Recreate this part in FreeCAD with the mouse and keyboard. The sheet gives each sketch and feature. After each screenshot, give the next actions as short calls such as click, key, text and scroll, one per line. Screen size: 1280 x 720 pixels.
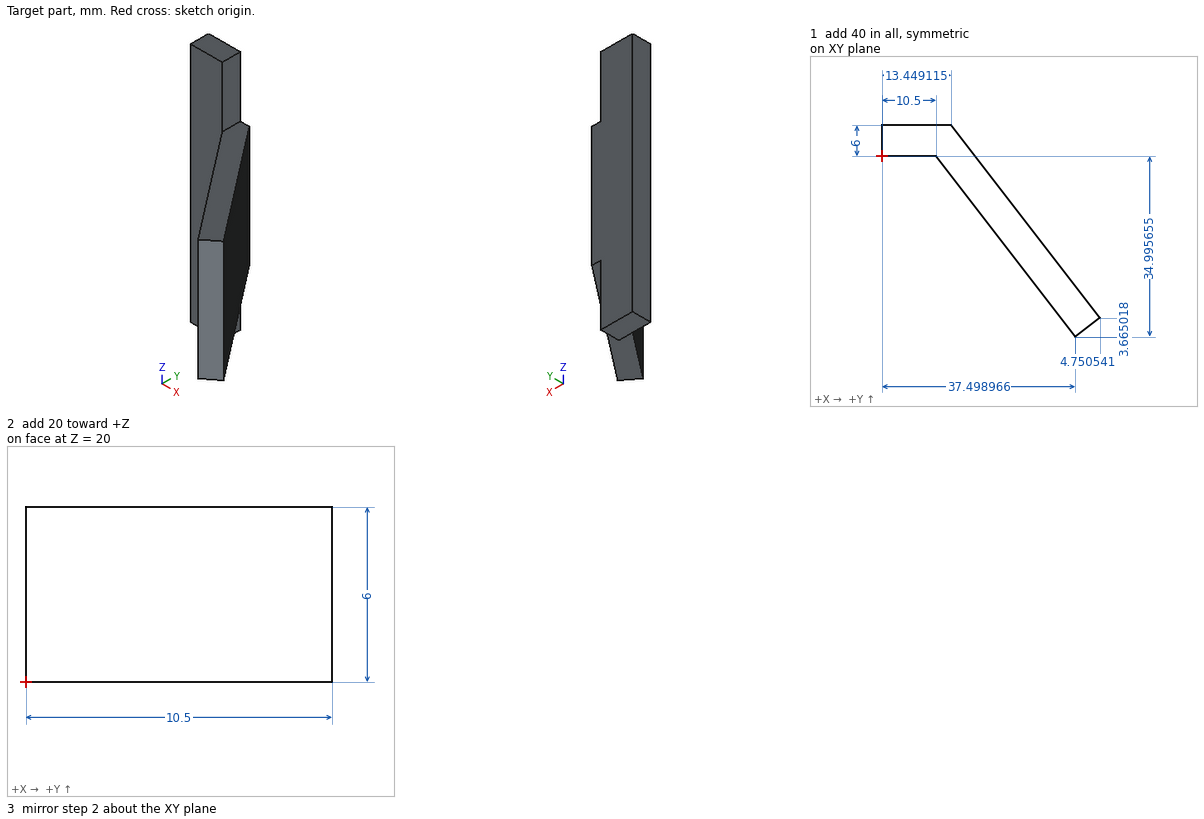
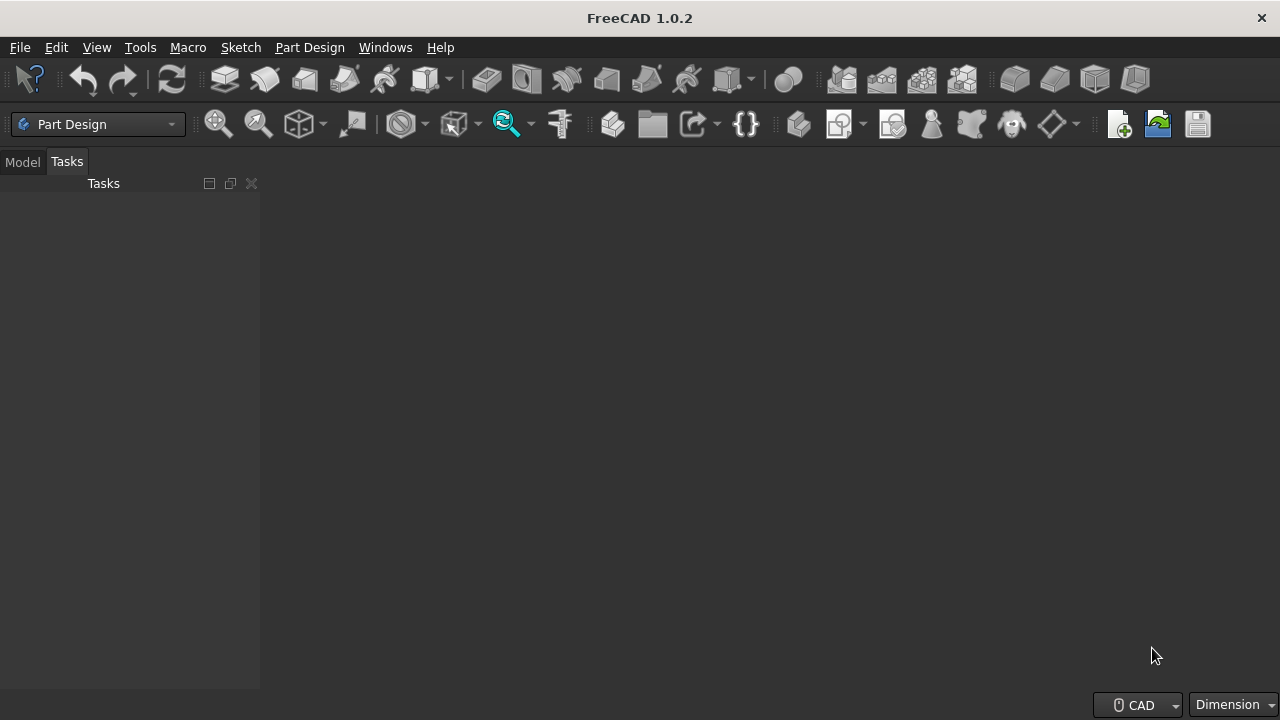
click(1118, 124)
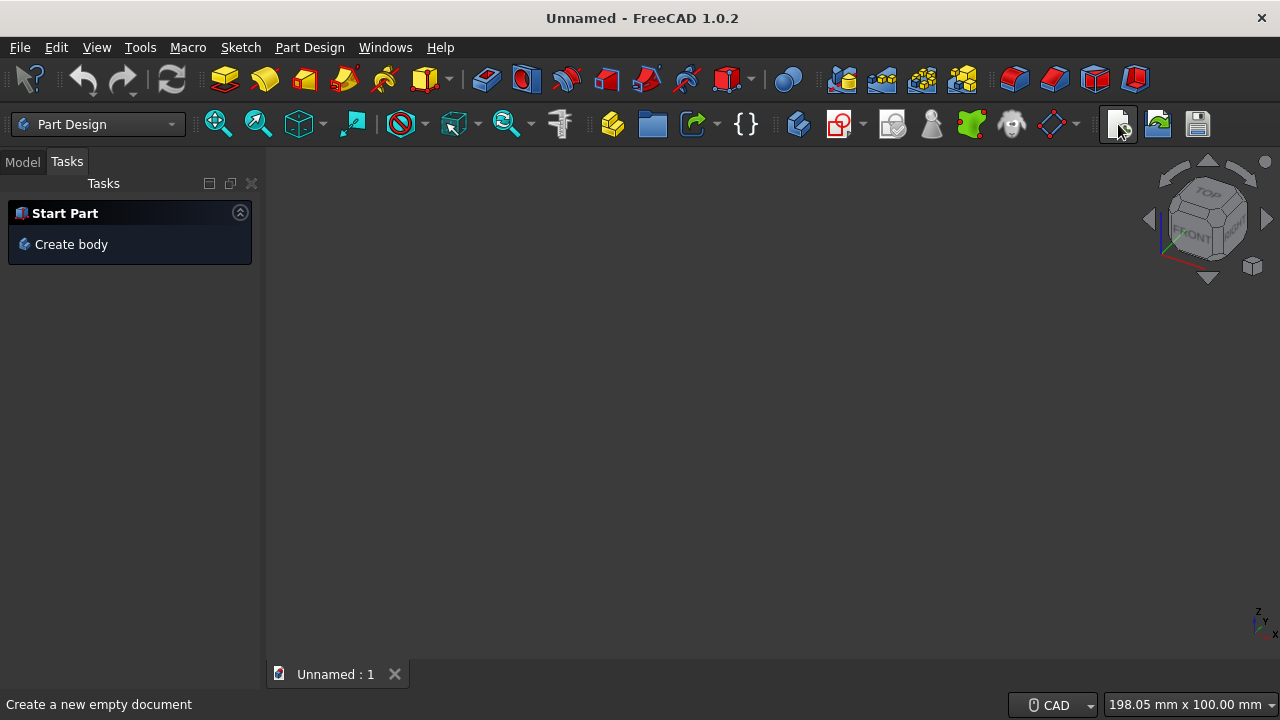
click(840, 124)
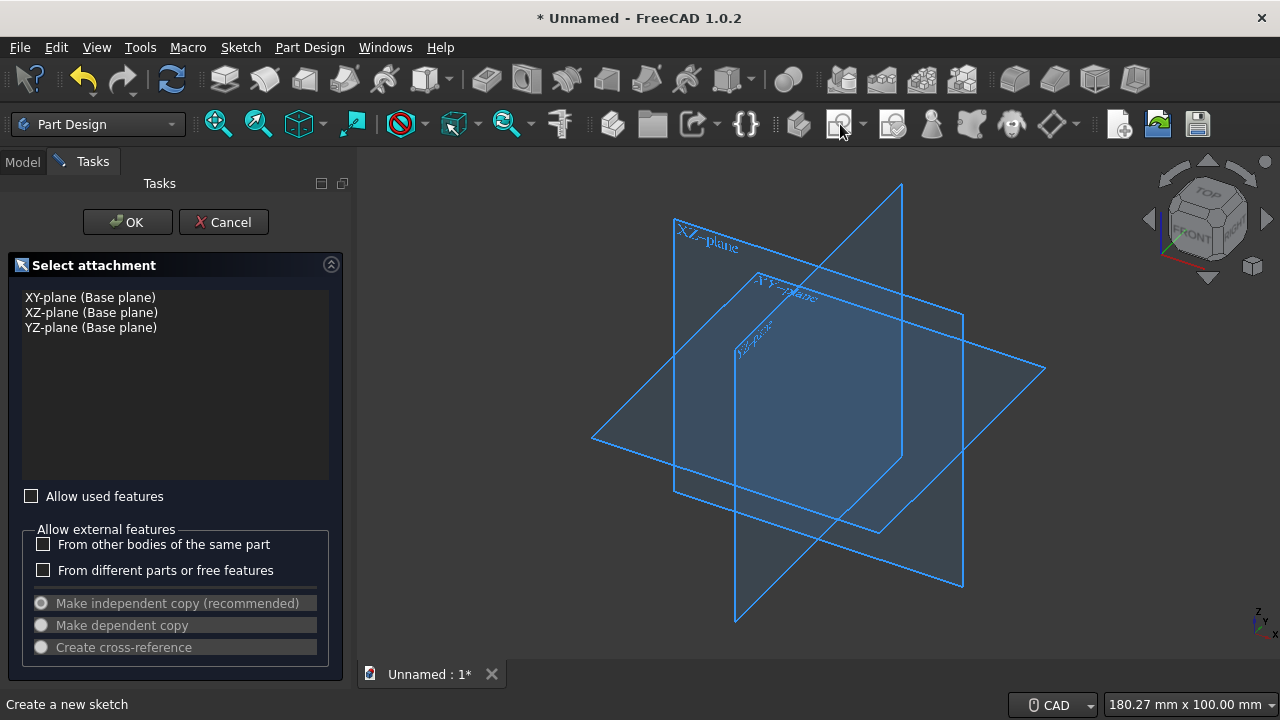
click(82, 298)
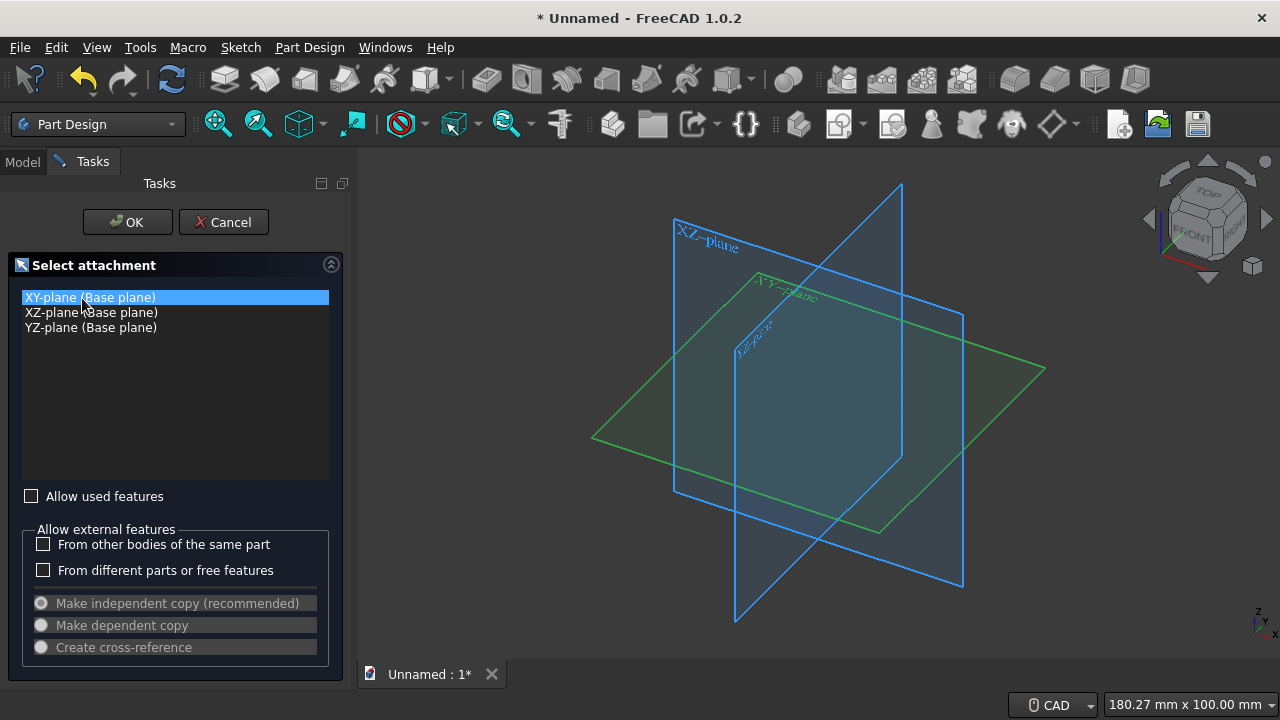
click(128, 222)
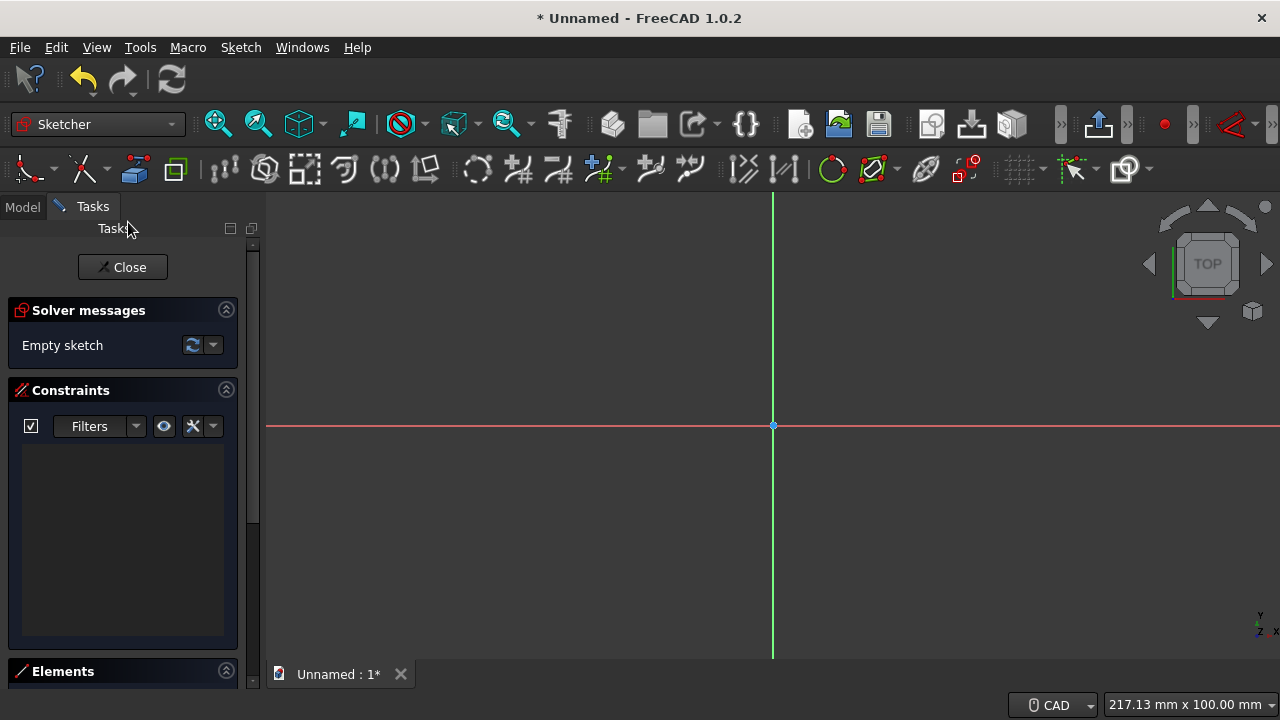
scroll(1115, 631, up, 2)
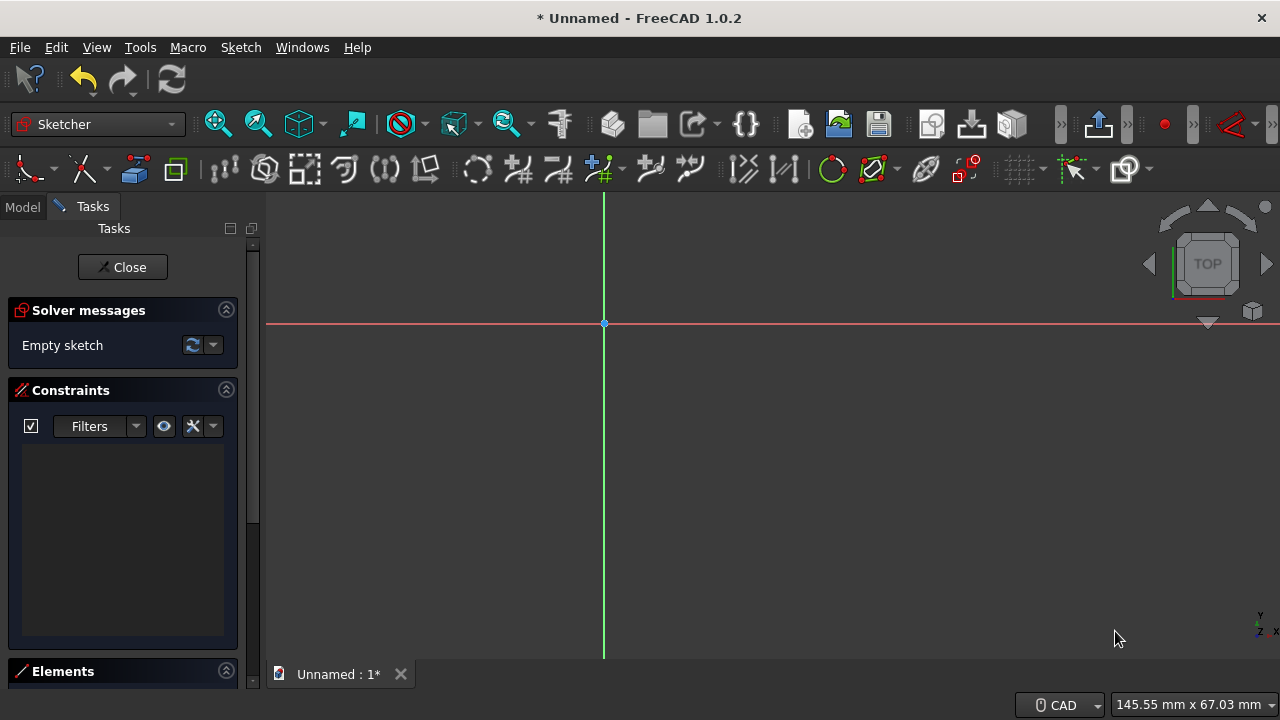
key(g)
key(m)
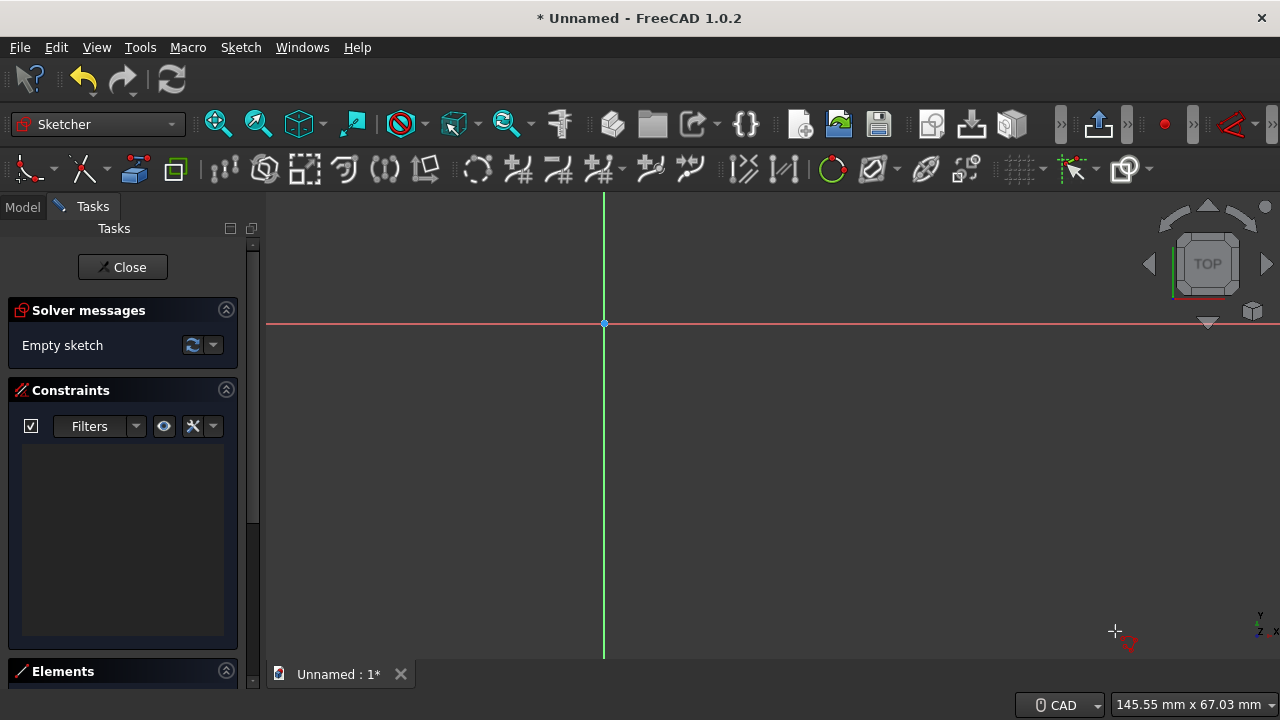
click(604, 324)
click(678, 333)
click(866, 568)
click(899, 542)
click(698, 282)
click(613, 282)
click(604, 324)
key(Escape)
key(Escape)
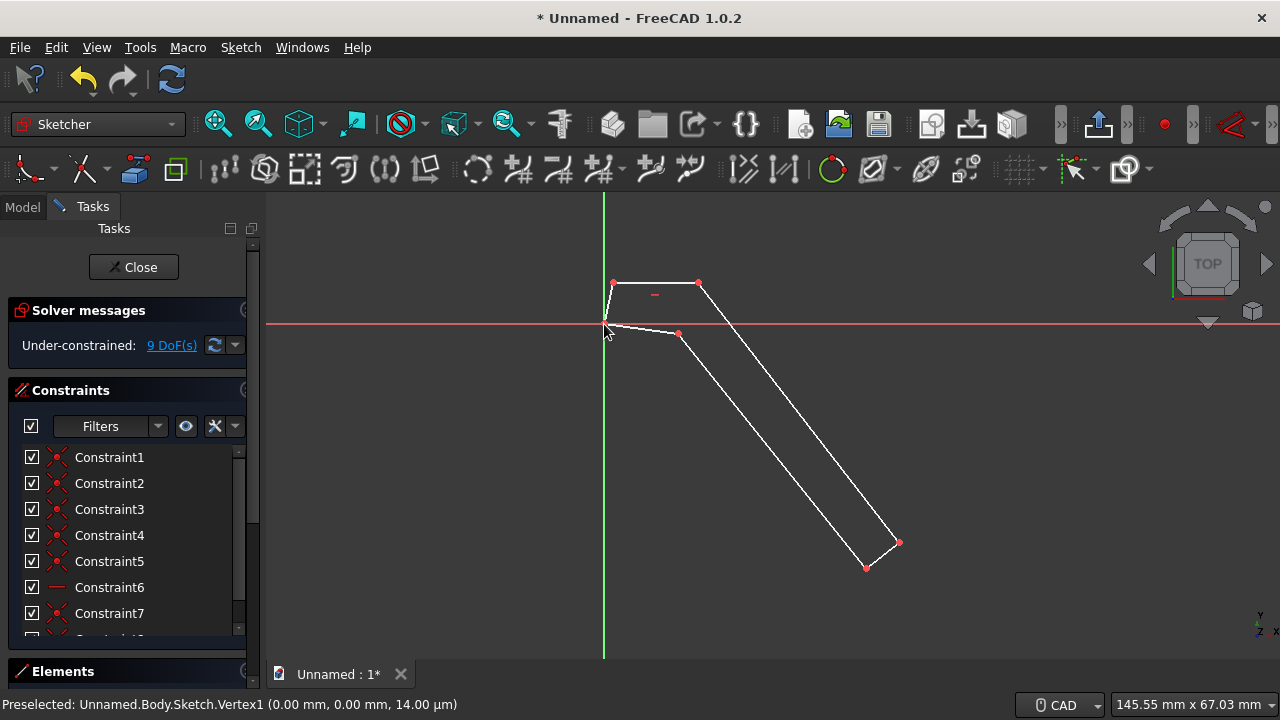
click(626, 327)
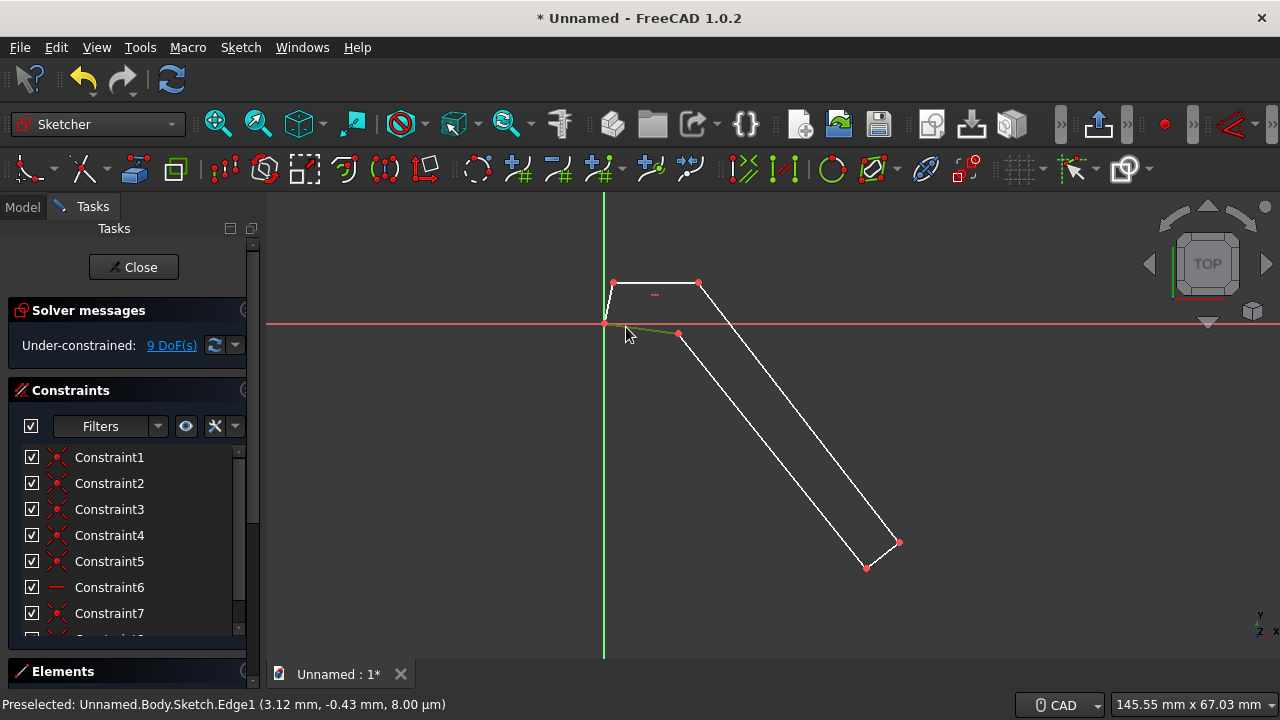
key(h)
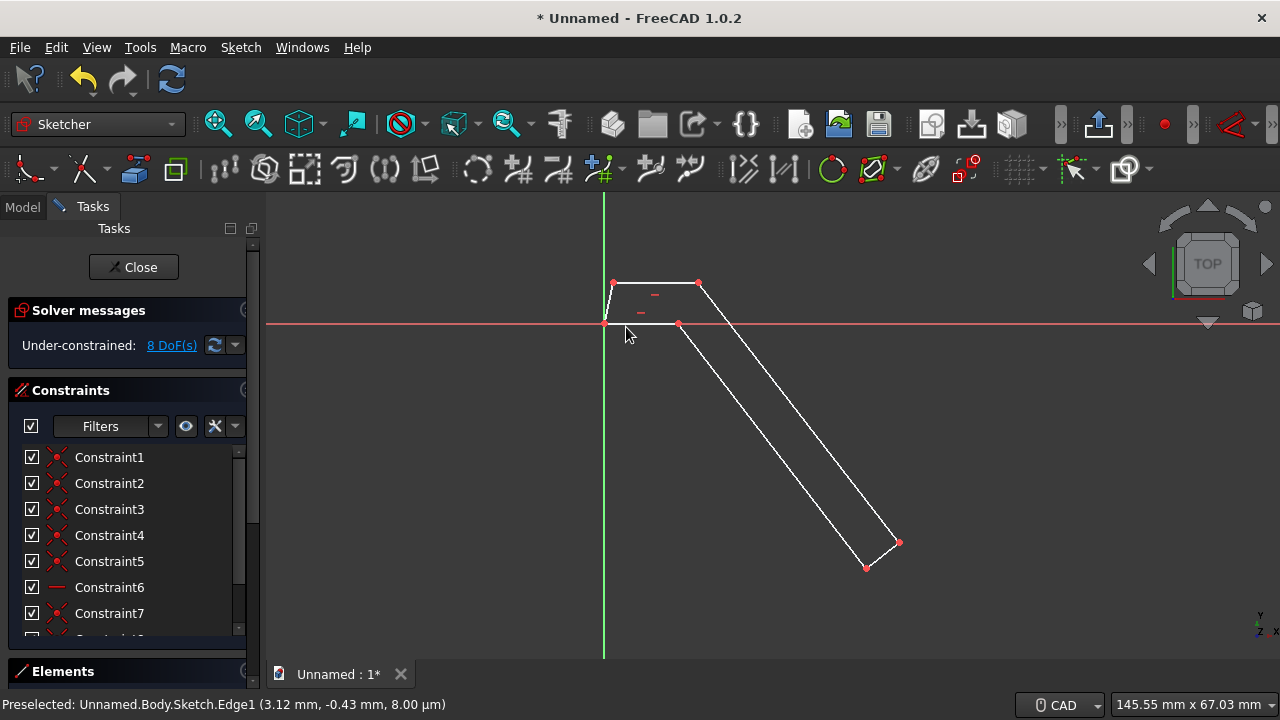
click(607, 312)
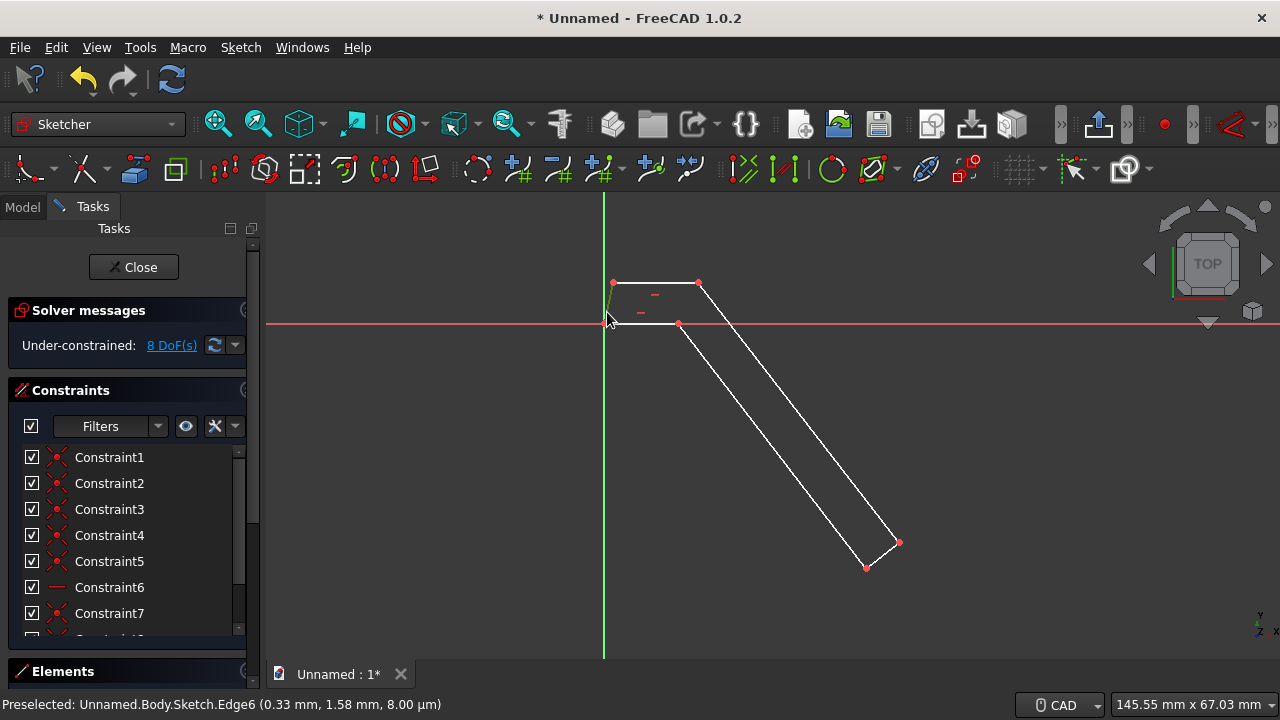
key(v)